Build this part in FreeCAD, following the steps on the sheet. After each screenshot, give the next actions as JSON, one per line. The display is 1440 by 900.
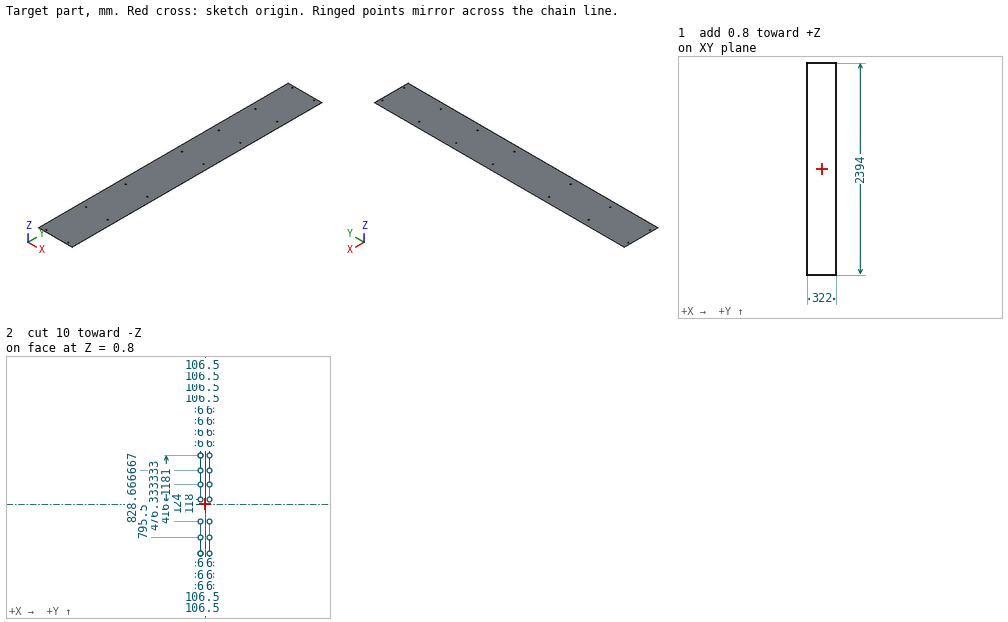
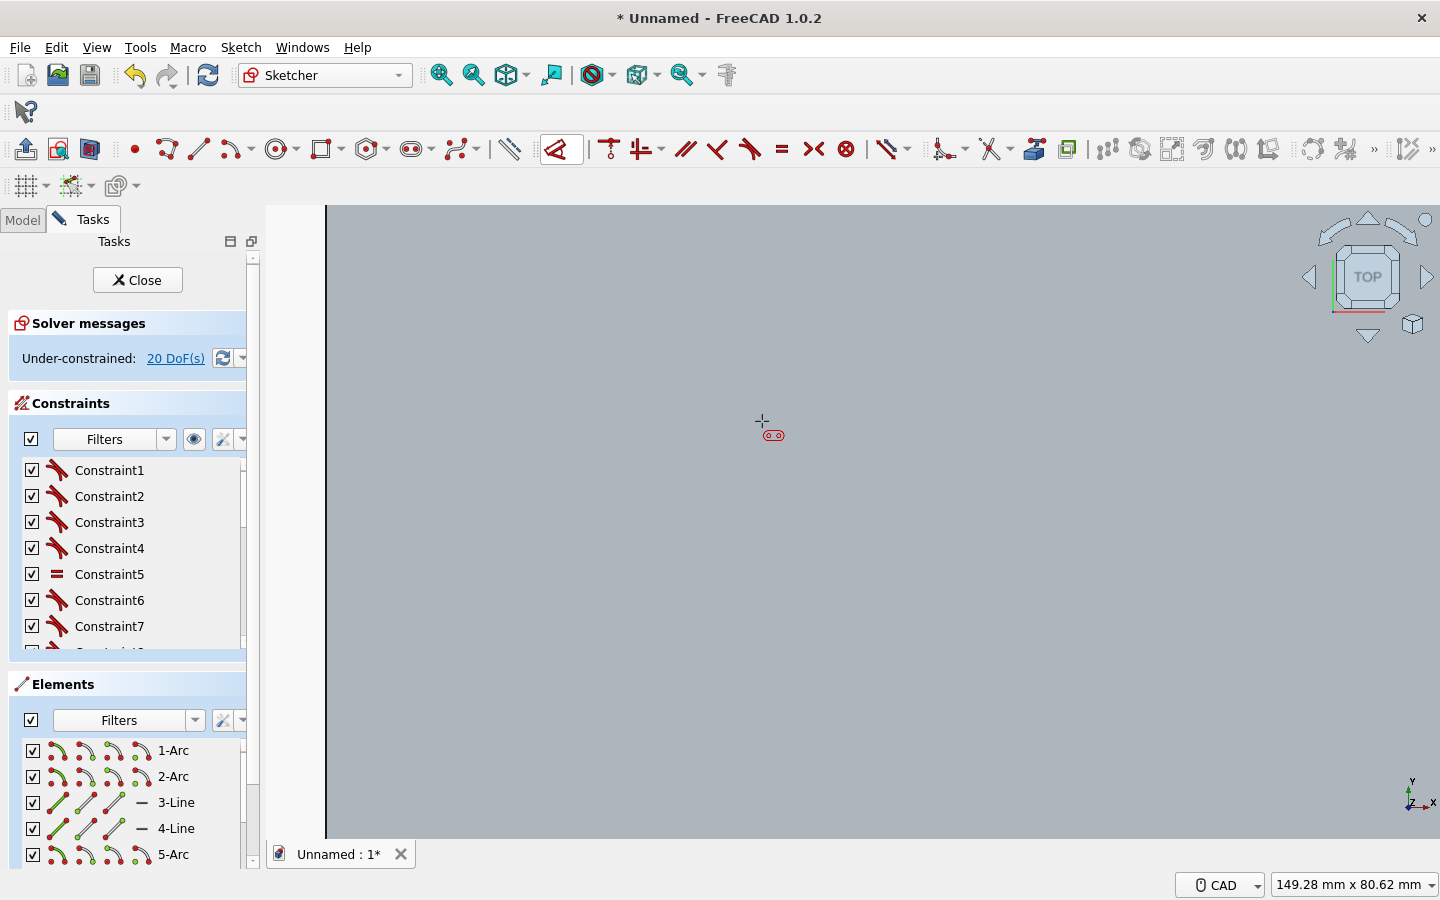
{"action": "scroll", "coordinate": [762, 421], "scroll_direction": "down", "scroll_amount": 18}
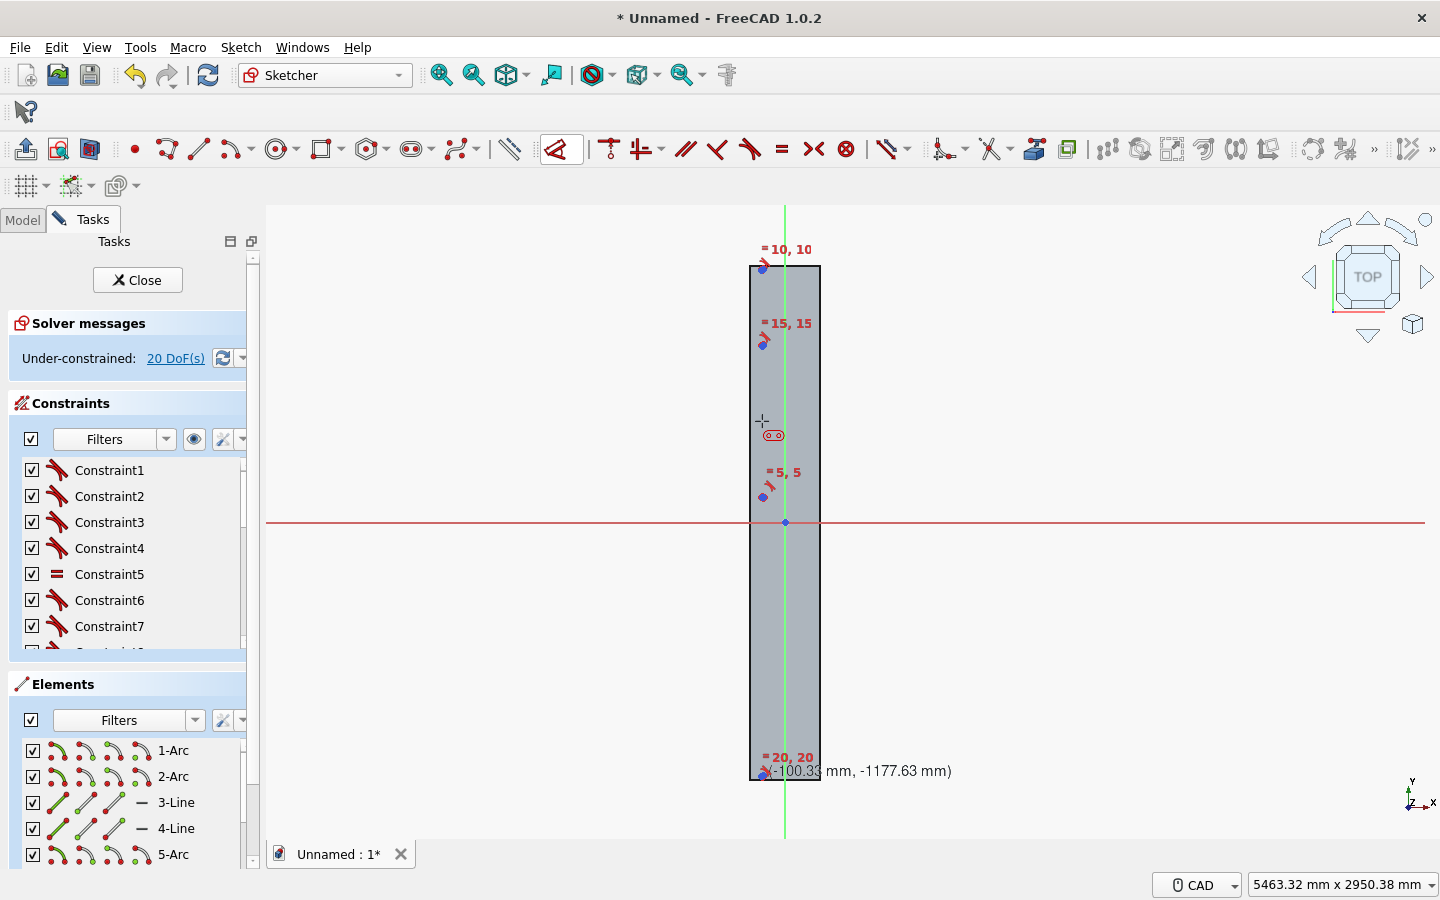
{"action": "left_click", "coordinate": [762, 421]}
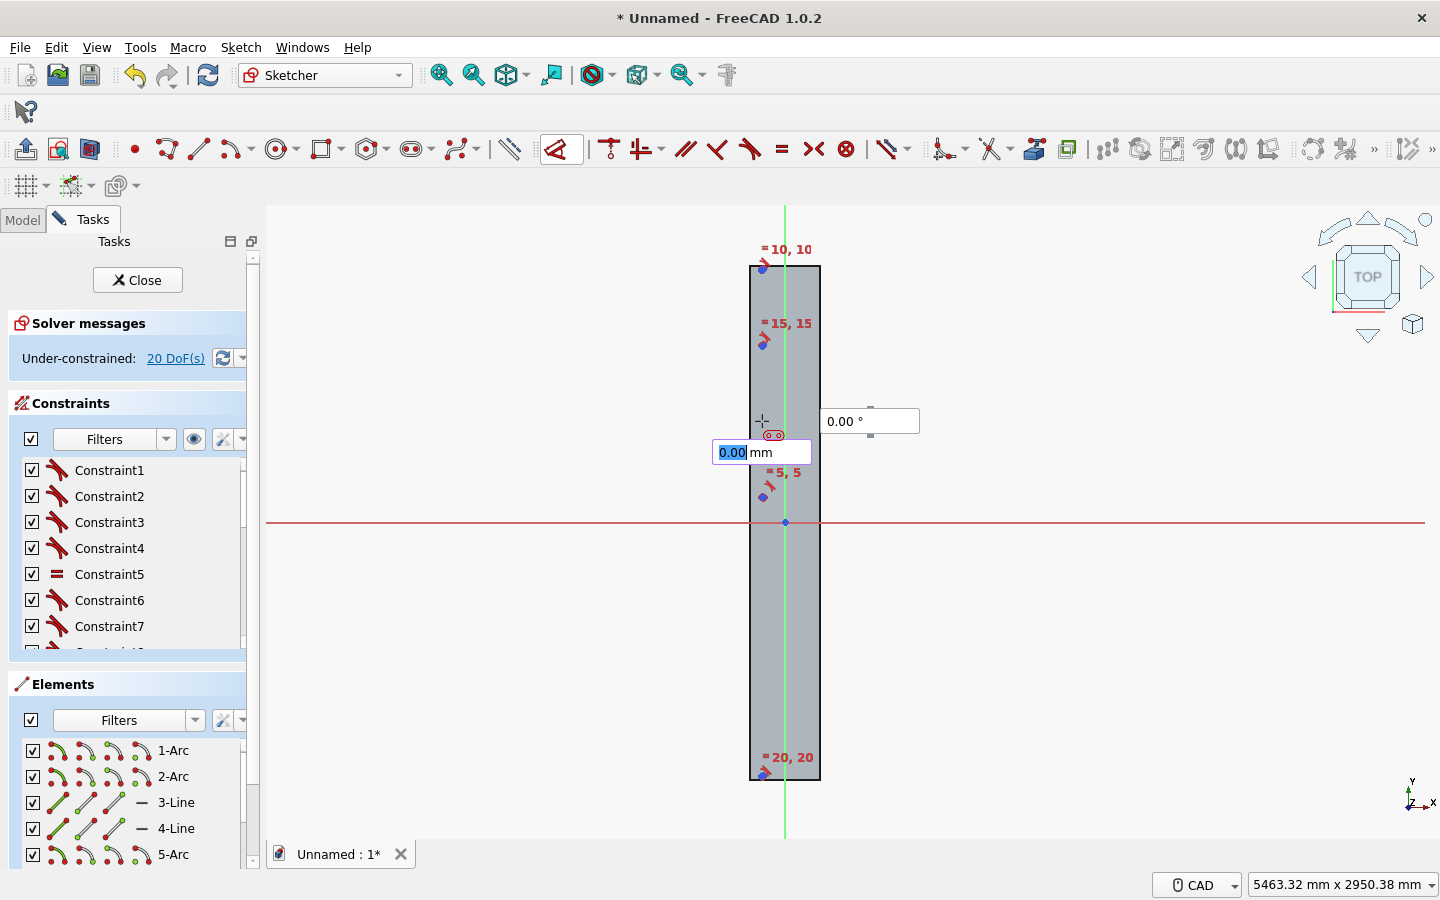
{"action": "scroll", "coordinate": [763, 421], "scroll_direction": "up", "scroll_amount": 13}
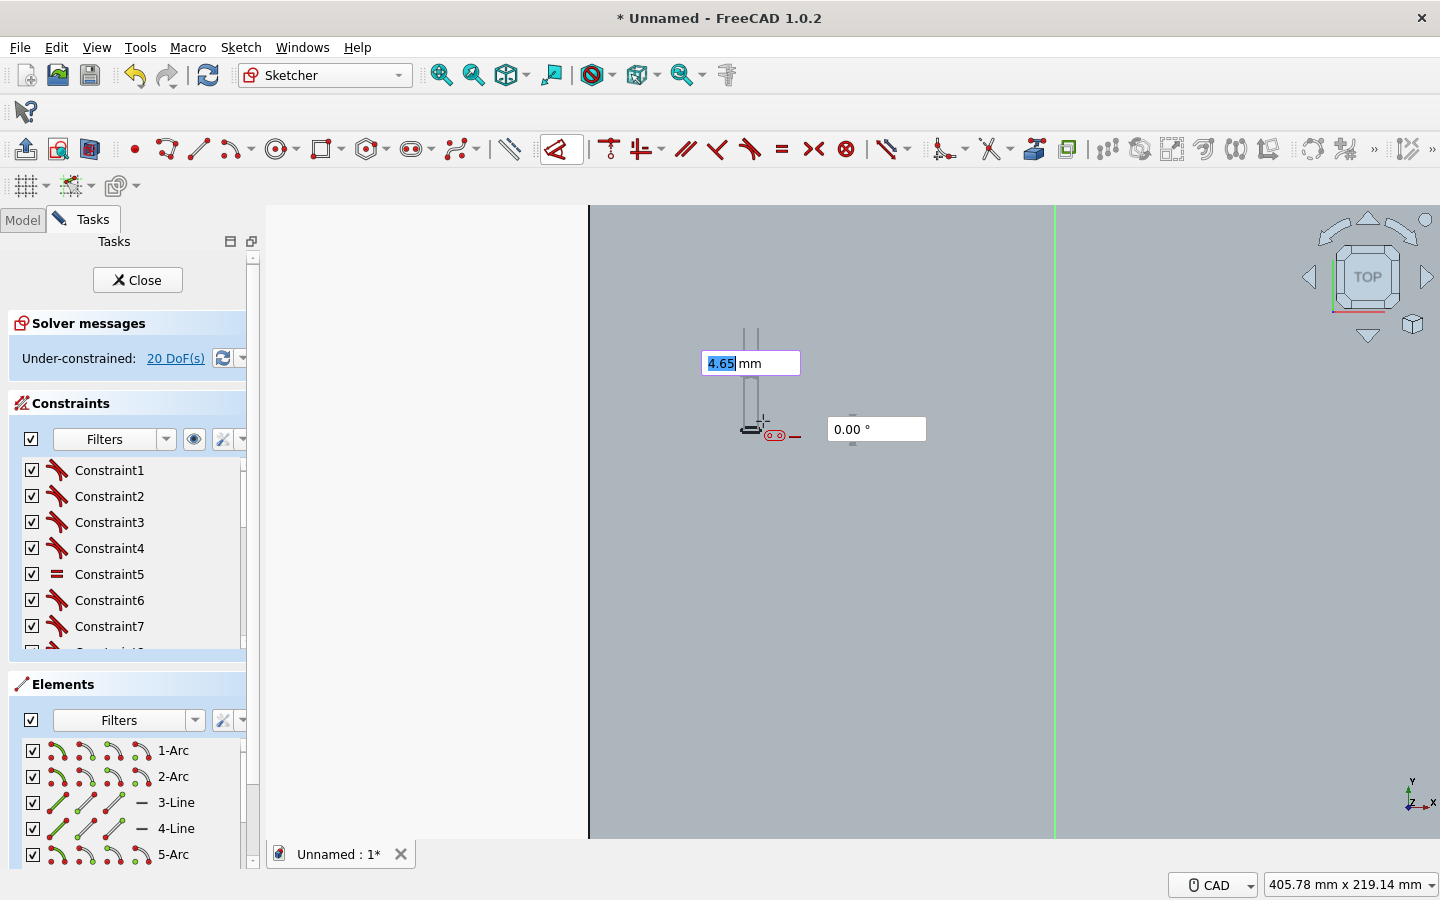
{"action": "left_click", "coordinate": [764, 417]}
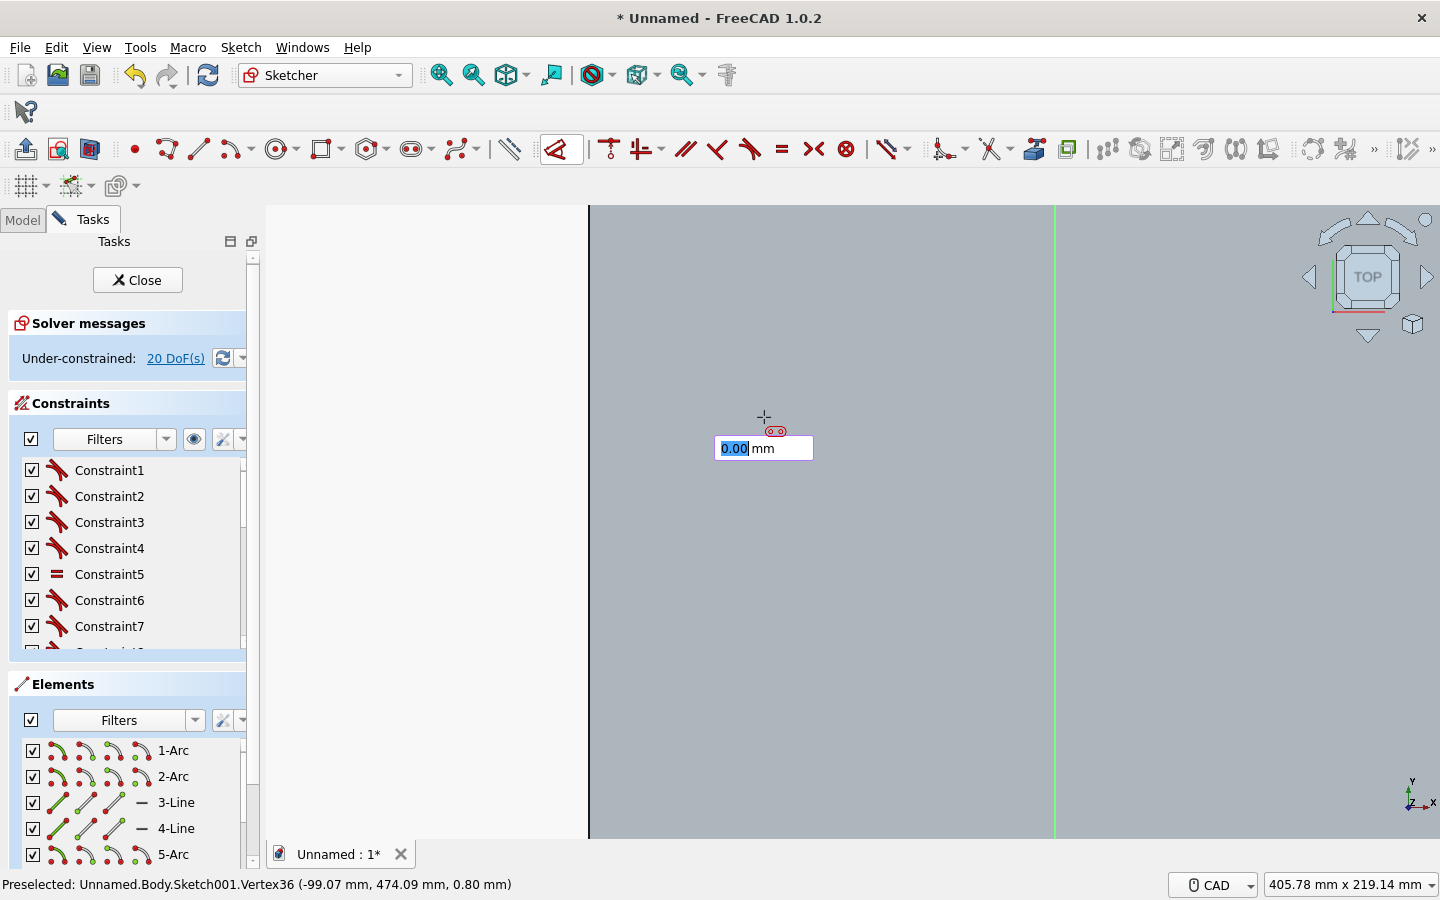
{"action": "scroll", "coordinate": [756, 409], "scroll_direction": "up", "scroll_amount": 4}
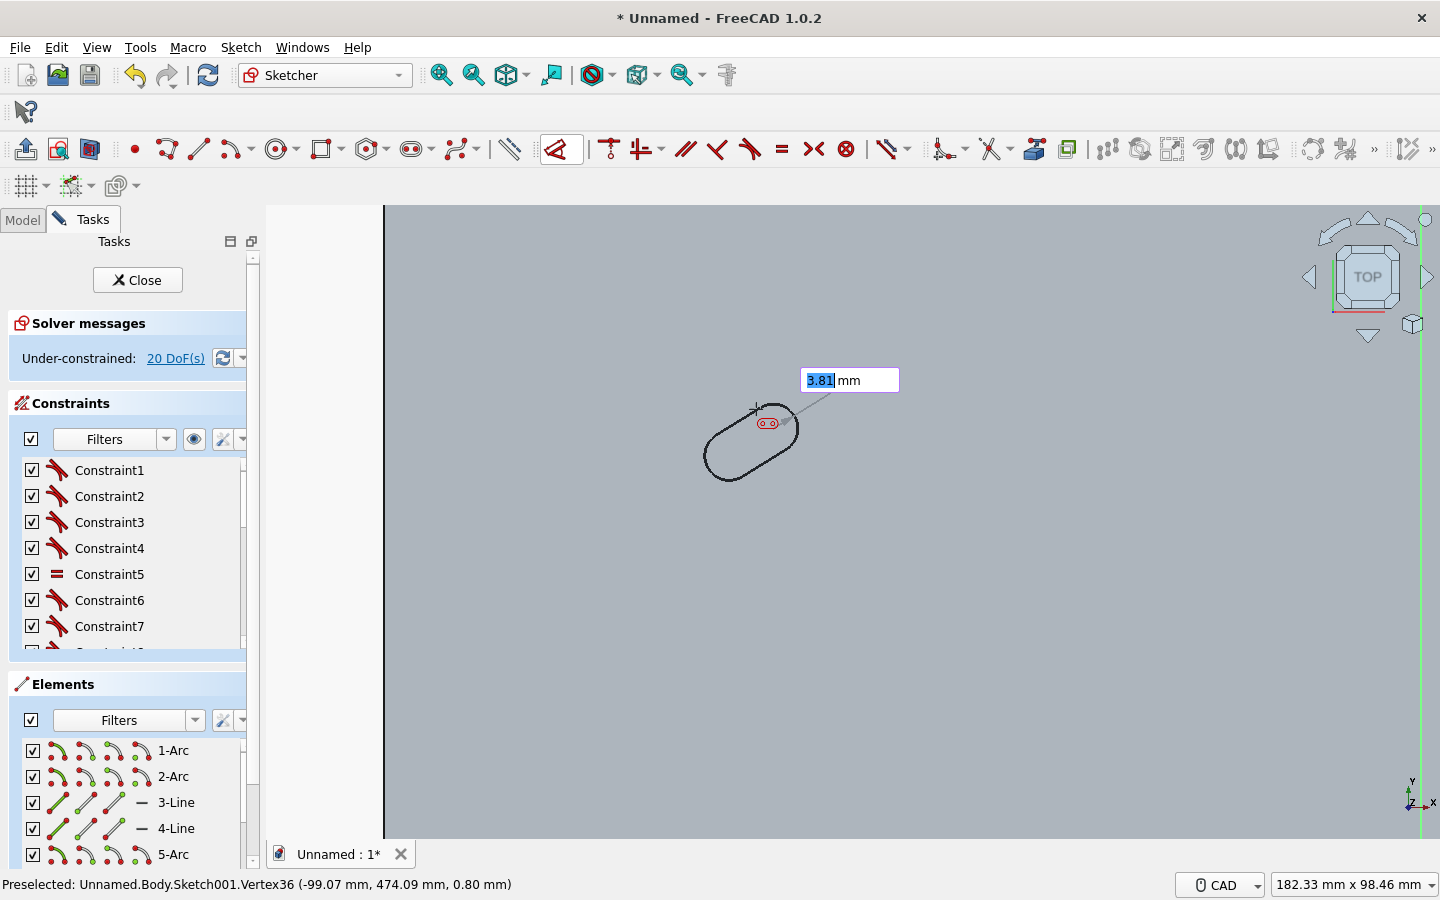
{"action": "left_click", "coordinate": [755, 409]}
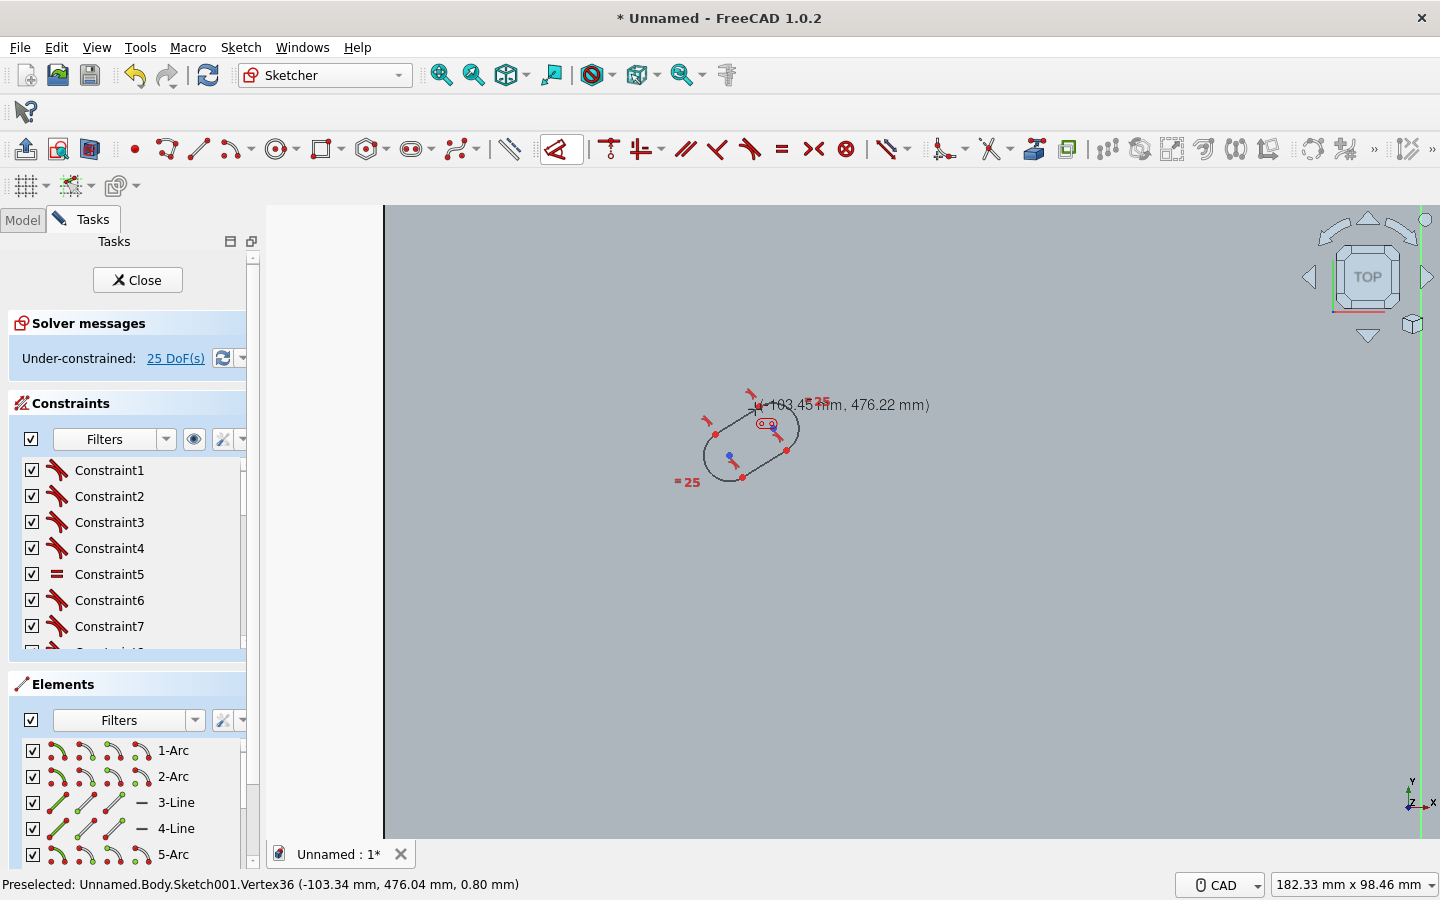
{"action": "scroll", "coordinate": [763, 420], "scroll_direction": "down", "scroll_amount": 17}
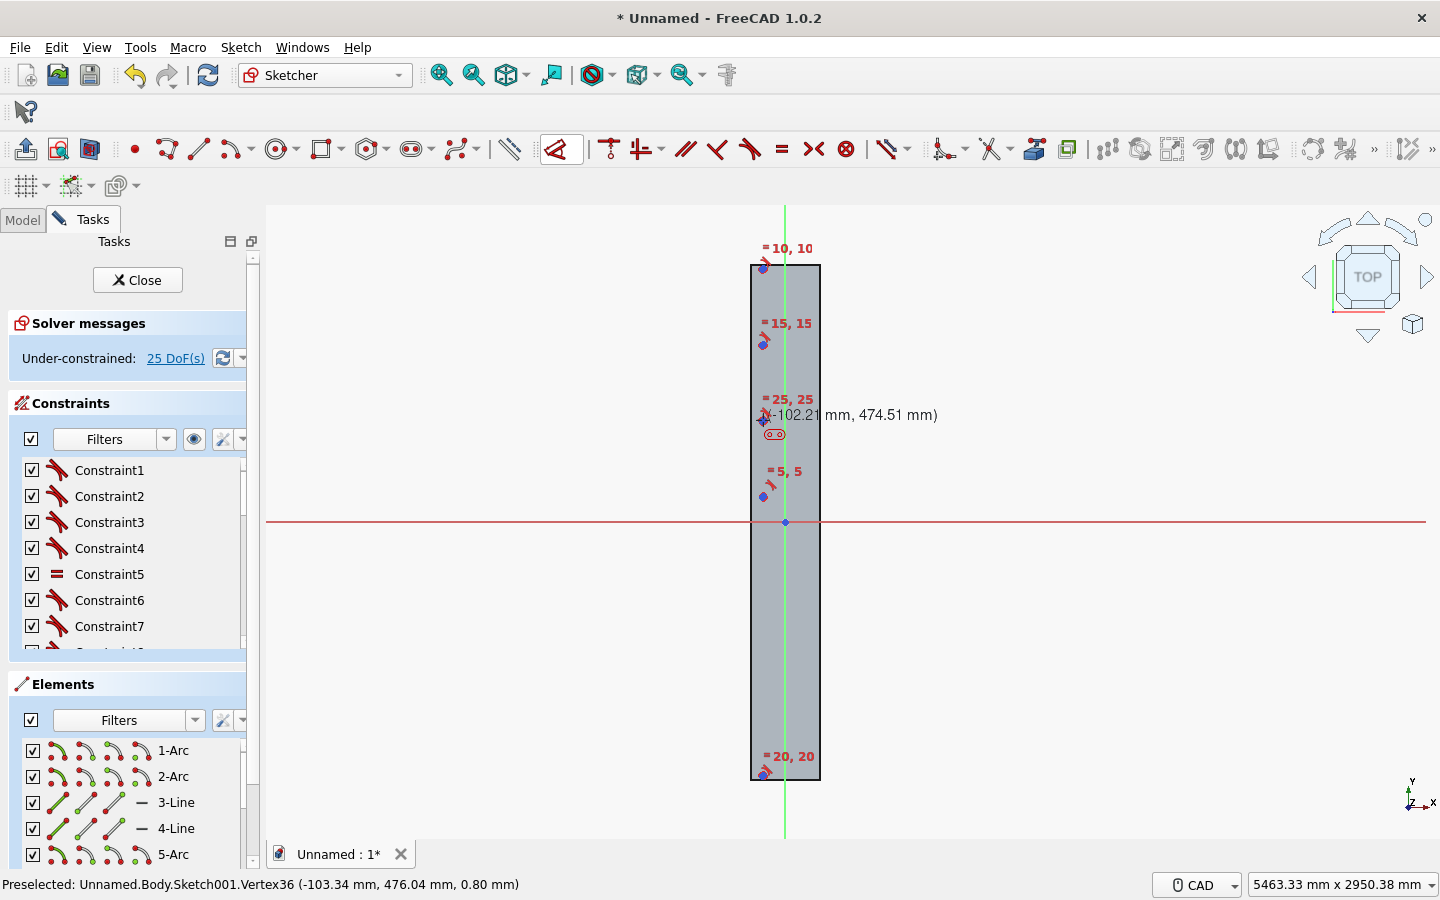
{"action": "scroll", "coordinate": [762, 694], "scroll_direction": "up", "scroll_amount": 18}